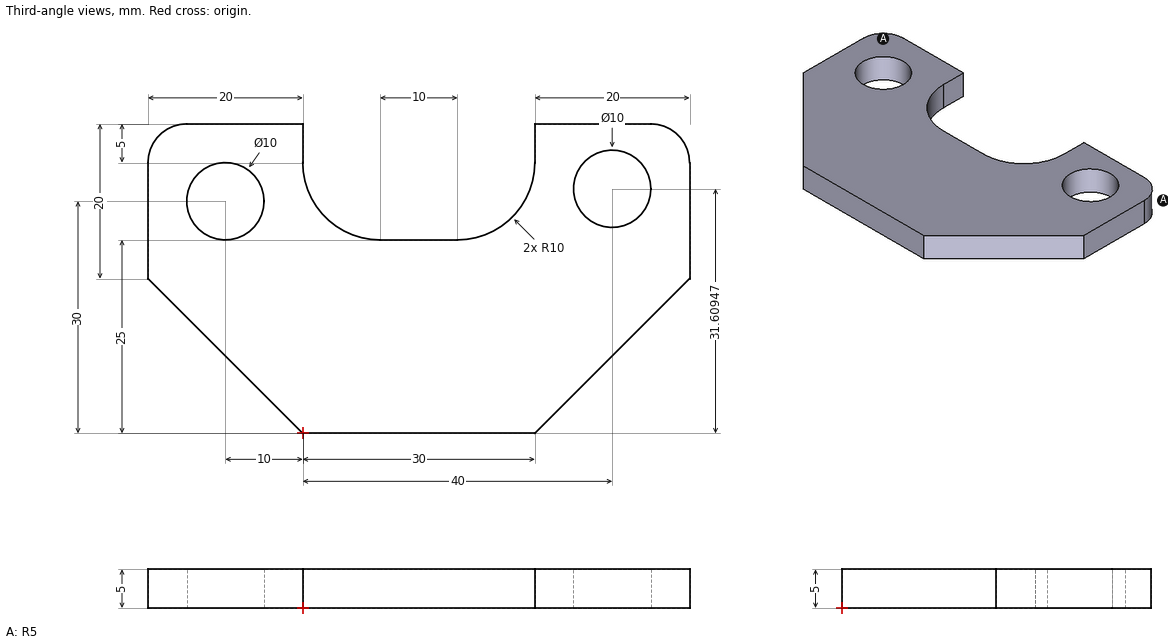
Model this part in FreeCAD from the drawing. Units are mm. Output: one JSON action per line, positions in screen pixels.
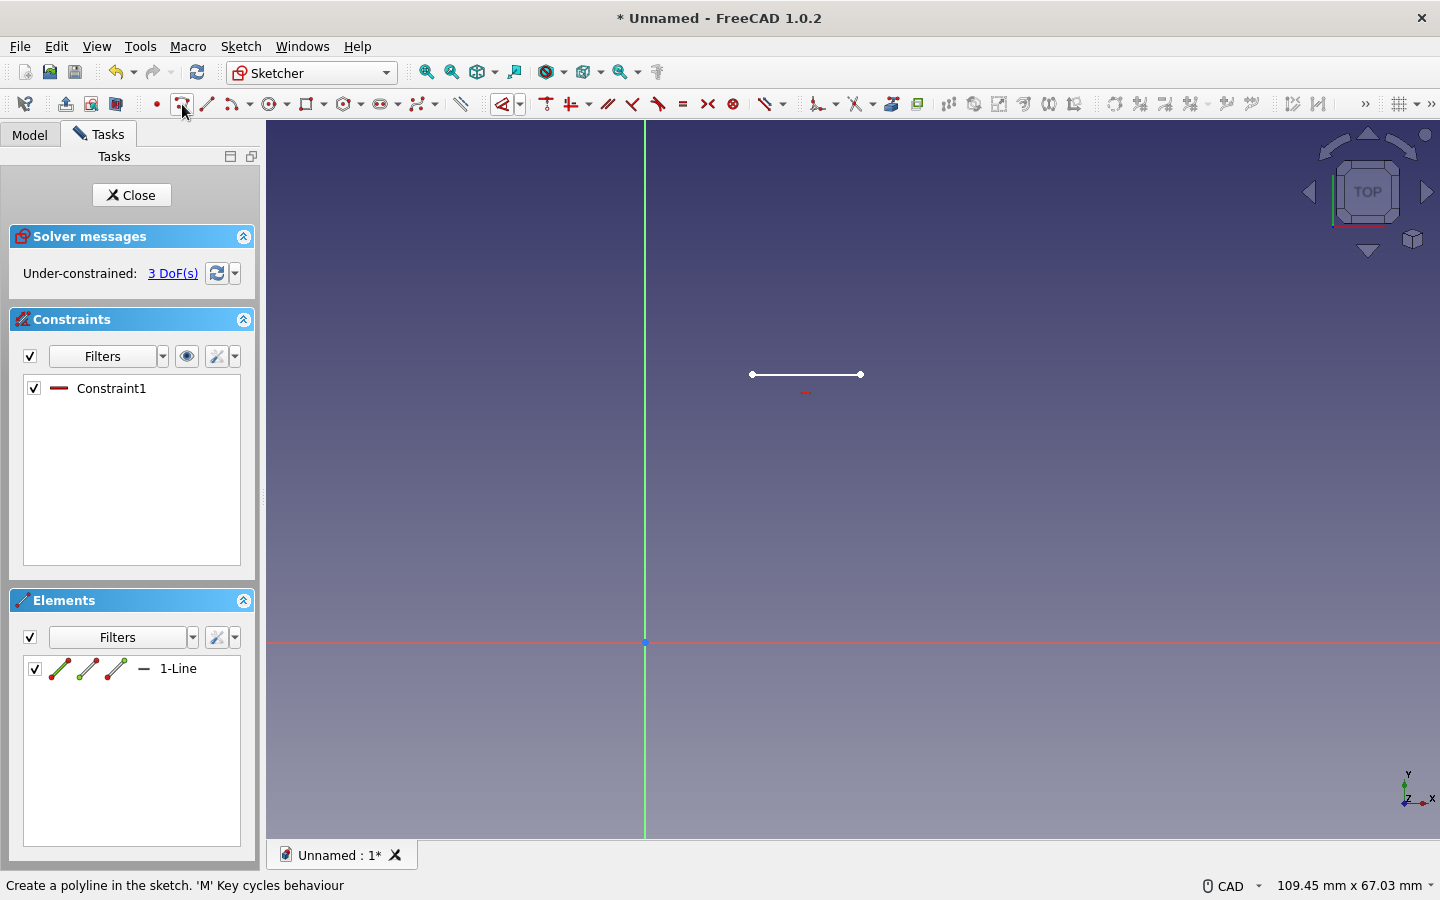
{"action": "left_click", "coordinate": [645, 267]}
{"action": "left_click", "coordinate": [654, 213]}
{"action": "left_click", "coordinate": [431, 213]}
{"action": "left_click", "coordinate": [431, 428]}
{"action": "left_click", "coordinate": [645, 643]}
{"action": "left_click", "coordinate": [967, 634]}
{"action": "left_click", "coordinate": [1181, 428]}
{"action": "left_click", "coordinate": [1181, 213]}
{"action": "left_click", "coordinate": [967, 213]}
{"action": "left_click", "coordinate": [967, 267]}
{"action": "right_click", "coordinate": [967, 267]}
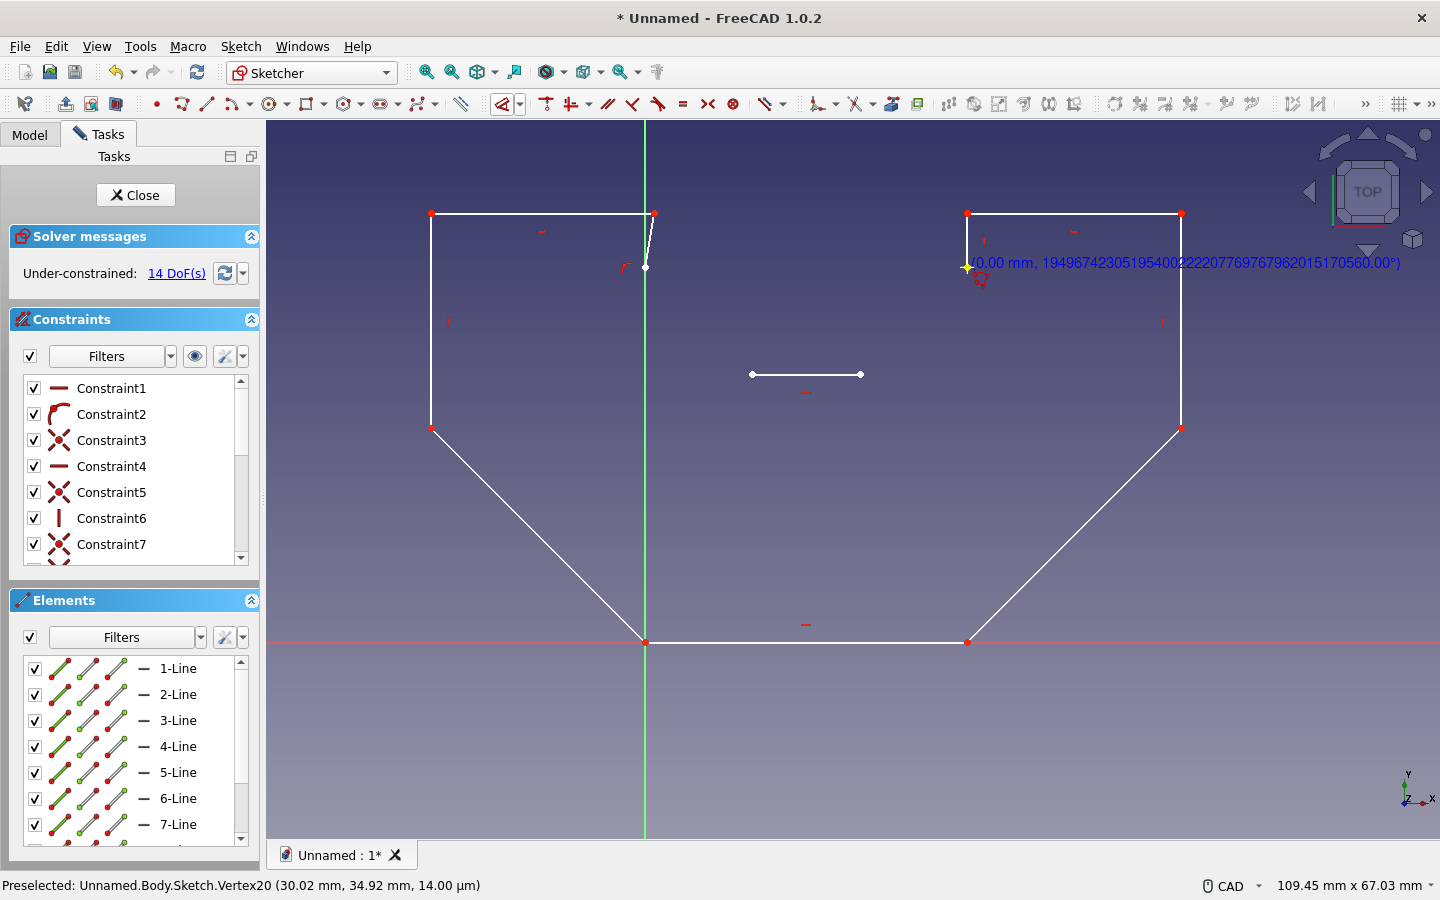
{"action": "left_click", "coordinate": [250, 104]}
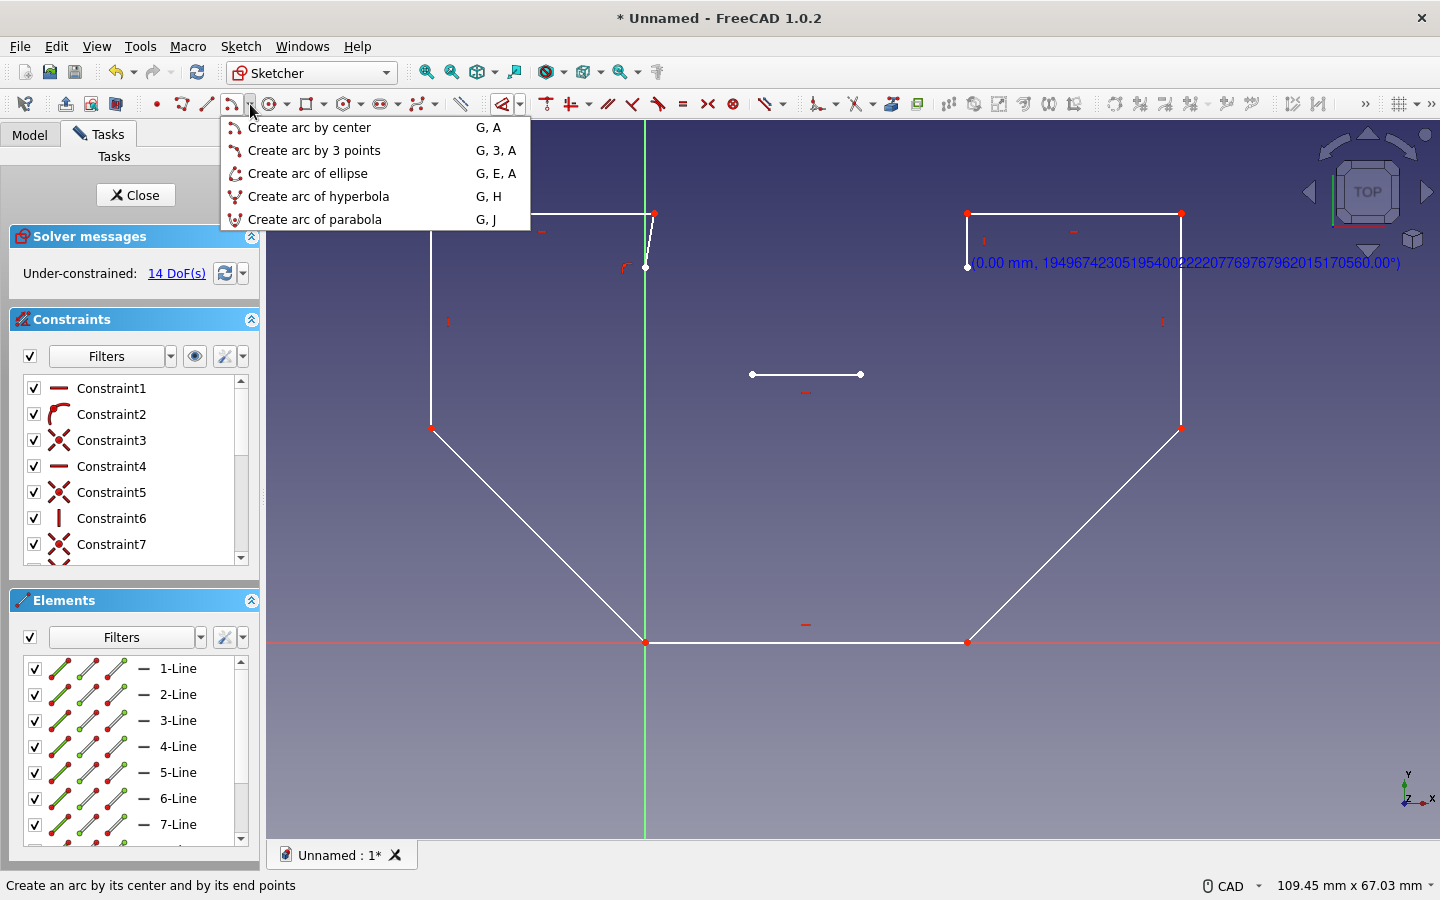
{"action": "left_click", "coordinate": [376, 150]}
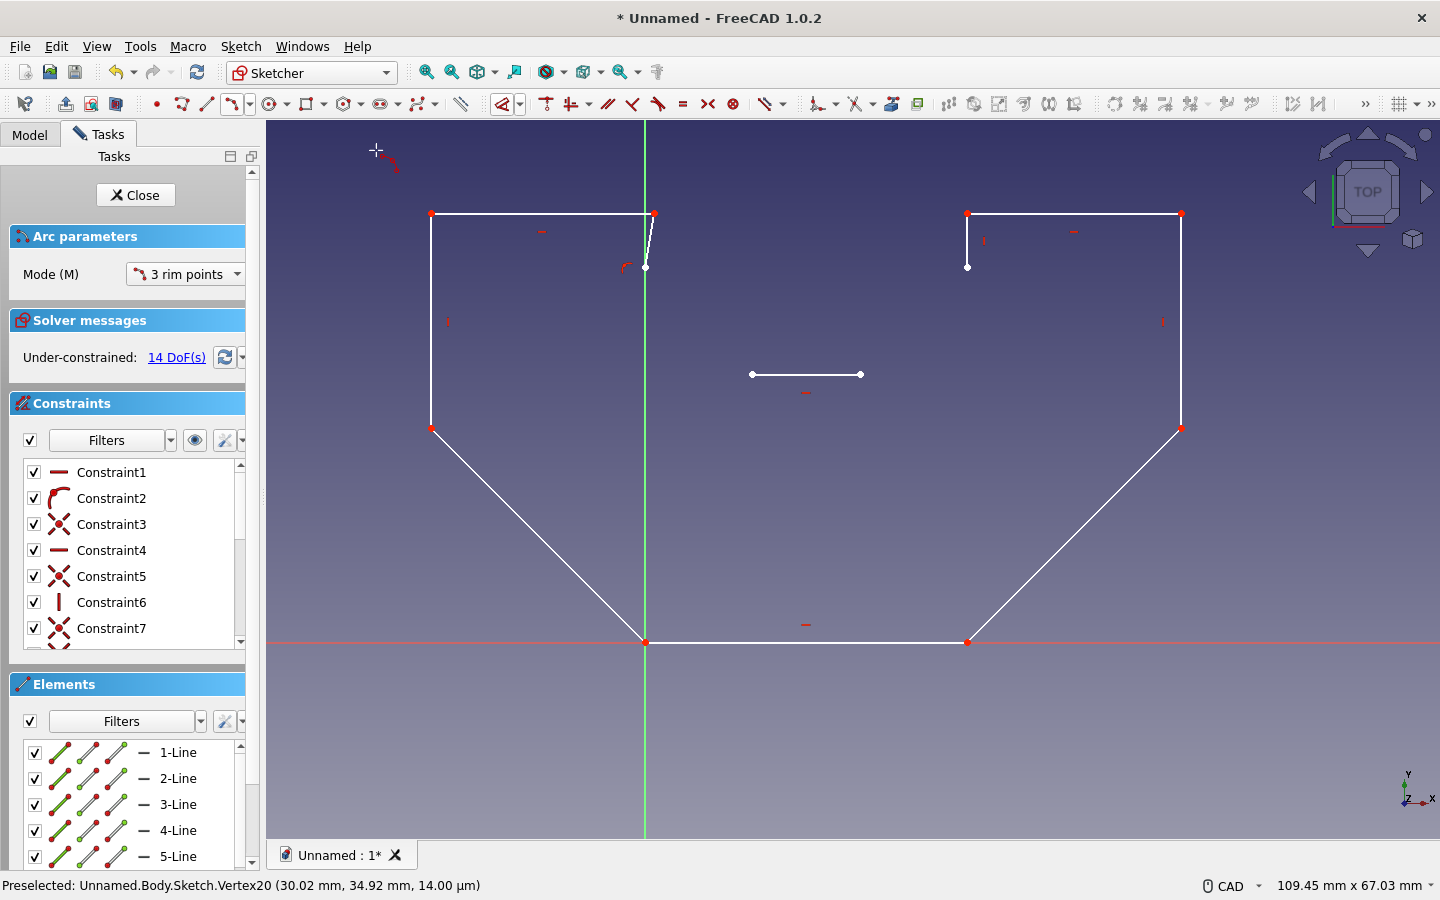
{"action": "left_click", "coordinate": [752, 375]}
{"action": "left_click", "coordinate": [645, 268]}
{"action": "left_click", "coordinate": [676, 343]}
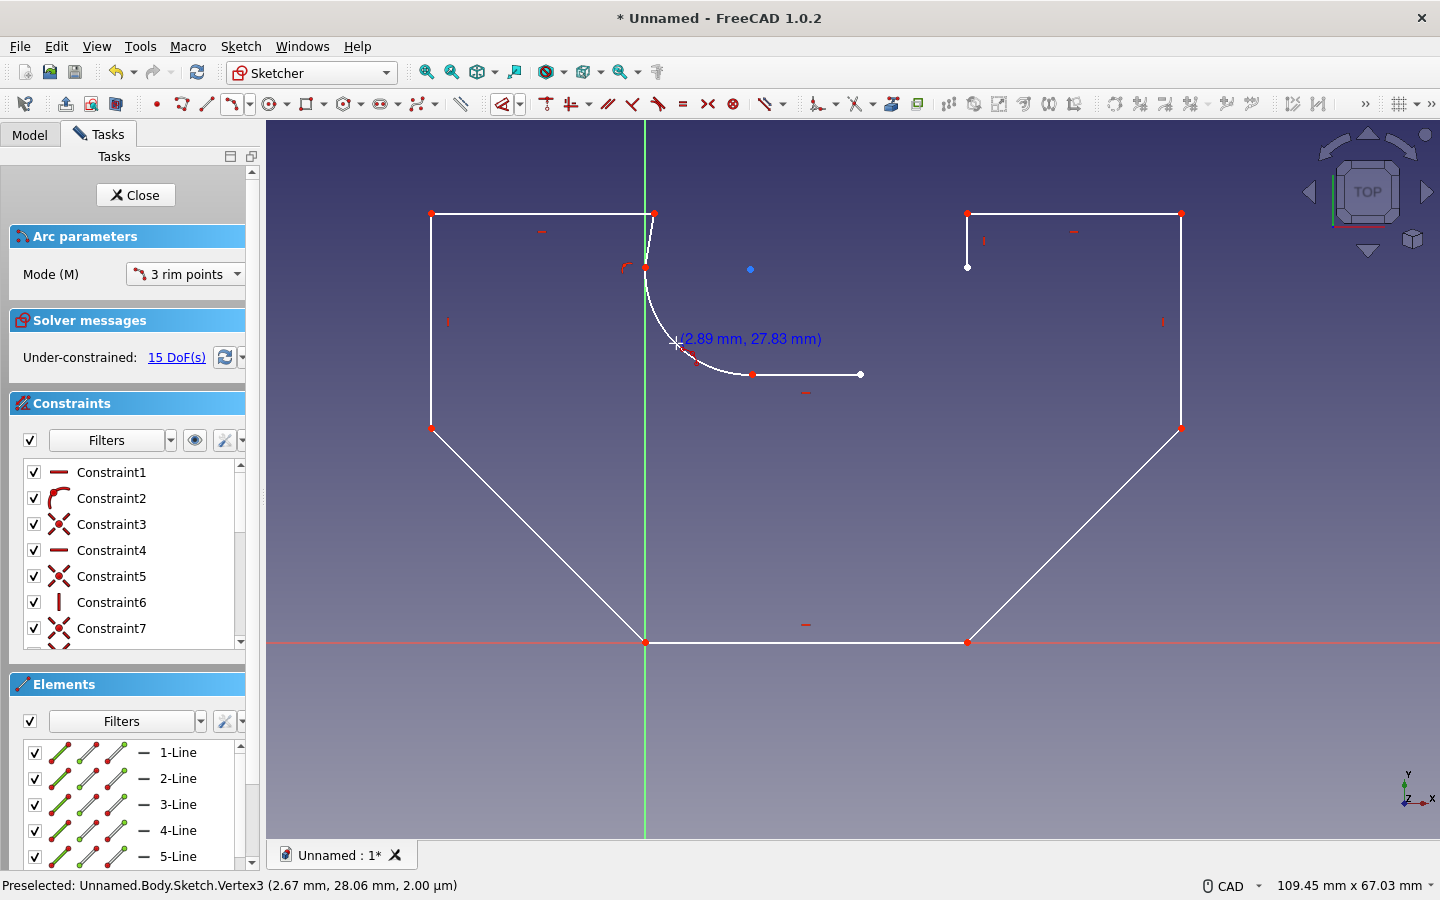
{"action": "left_click", "coordinate": [967, 268]}
{"action": "left_click", "coordinate": [860, 375]}
{"action": "left_click", "coordinate": [935, 343]}
{"action": "key", "text": "Escape"}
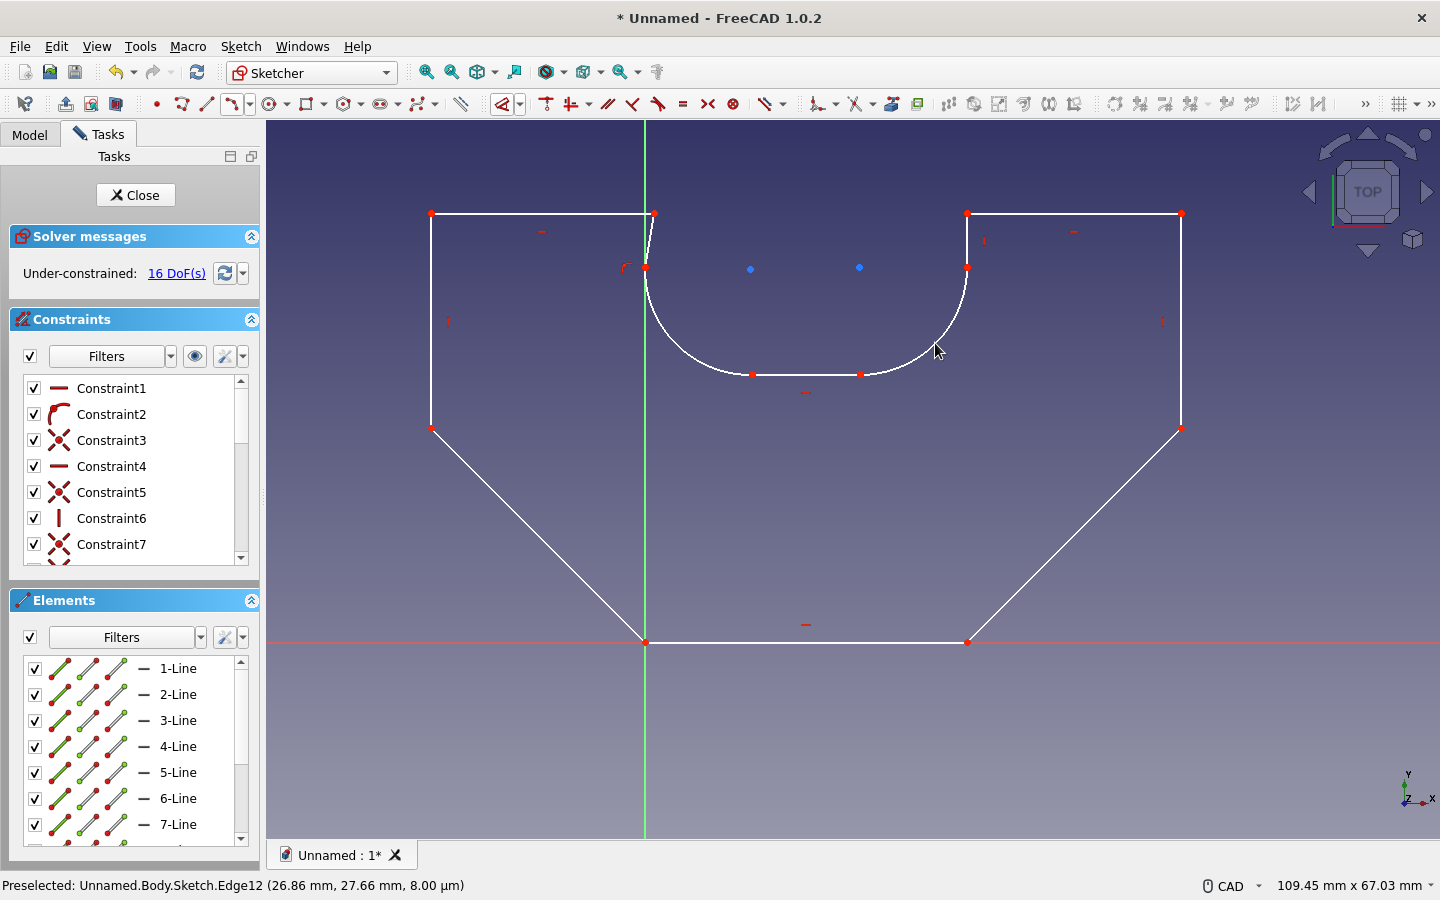
{"action": "left_click", "coordinate": [828, 375]}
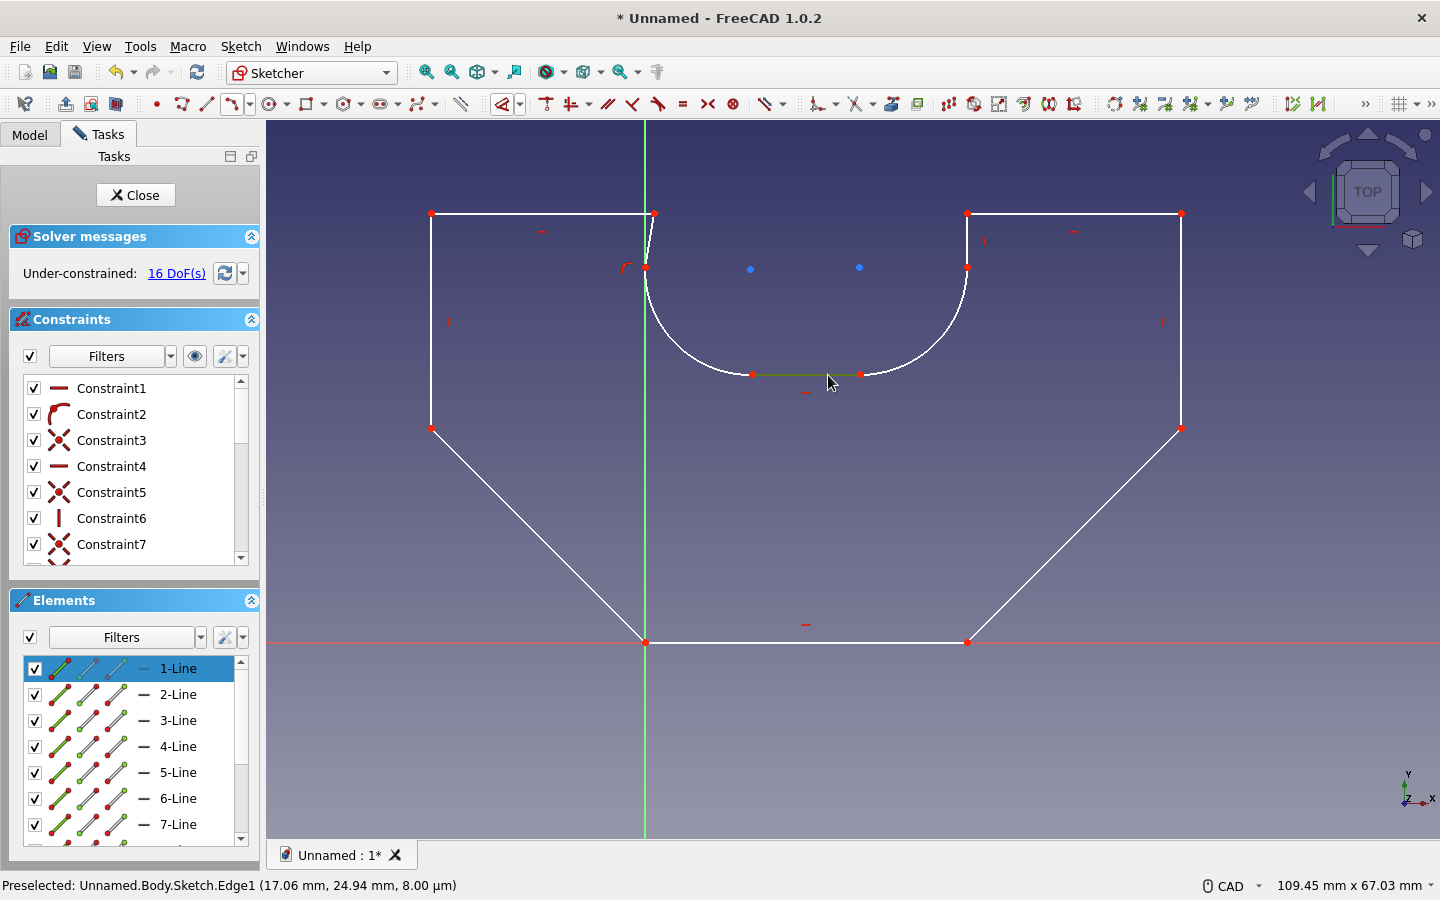
{"action": "left_click", "coordinate": [656, 317]}